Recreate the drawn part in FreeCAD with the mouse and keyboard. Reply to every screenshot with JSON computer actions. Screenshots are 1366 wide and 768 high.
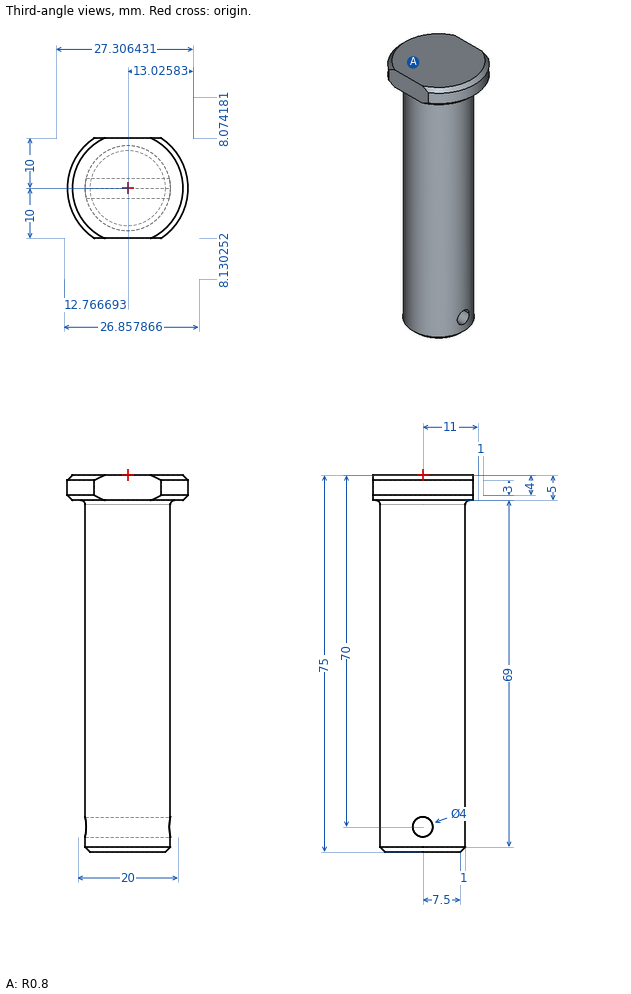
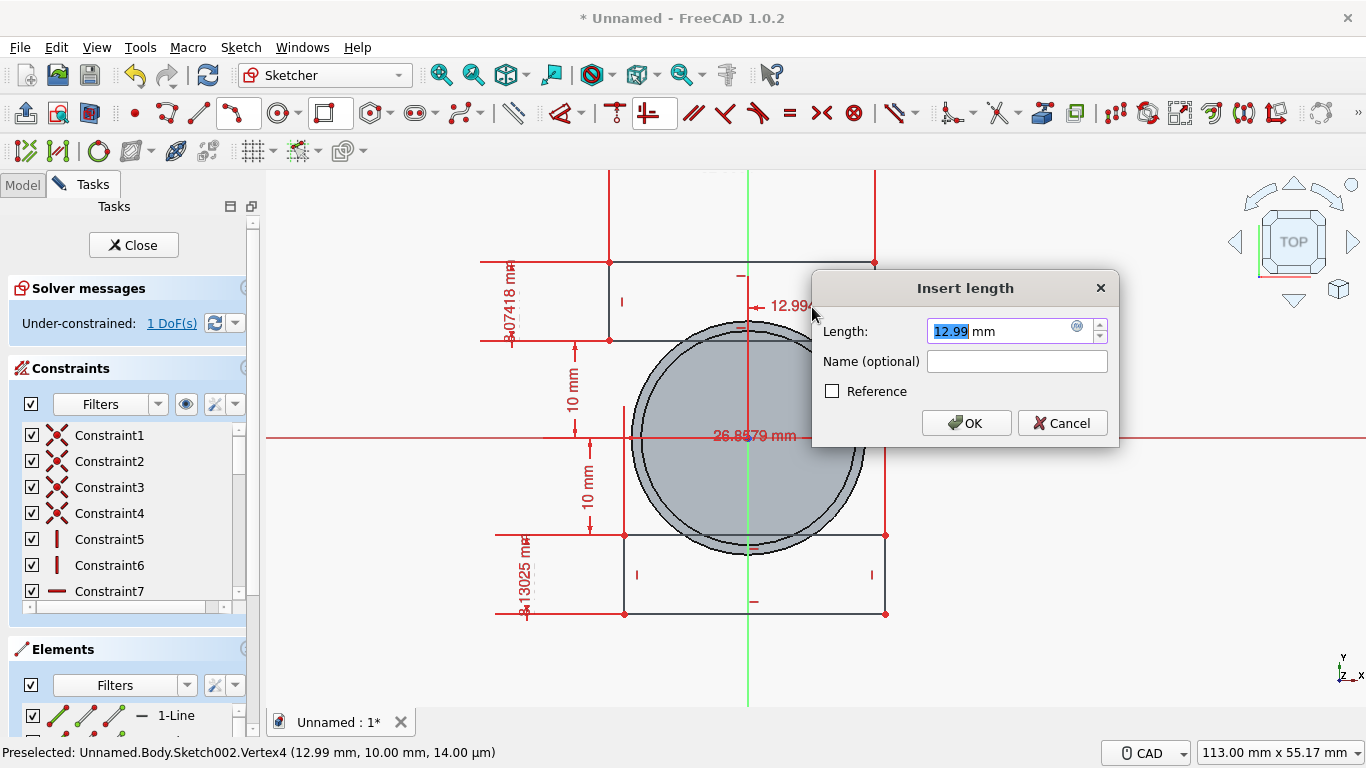
{"action": "type", "text": "13.02583"}
{"action": "key", "text": "Return"}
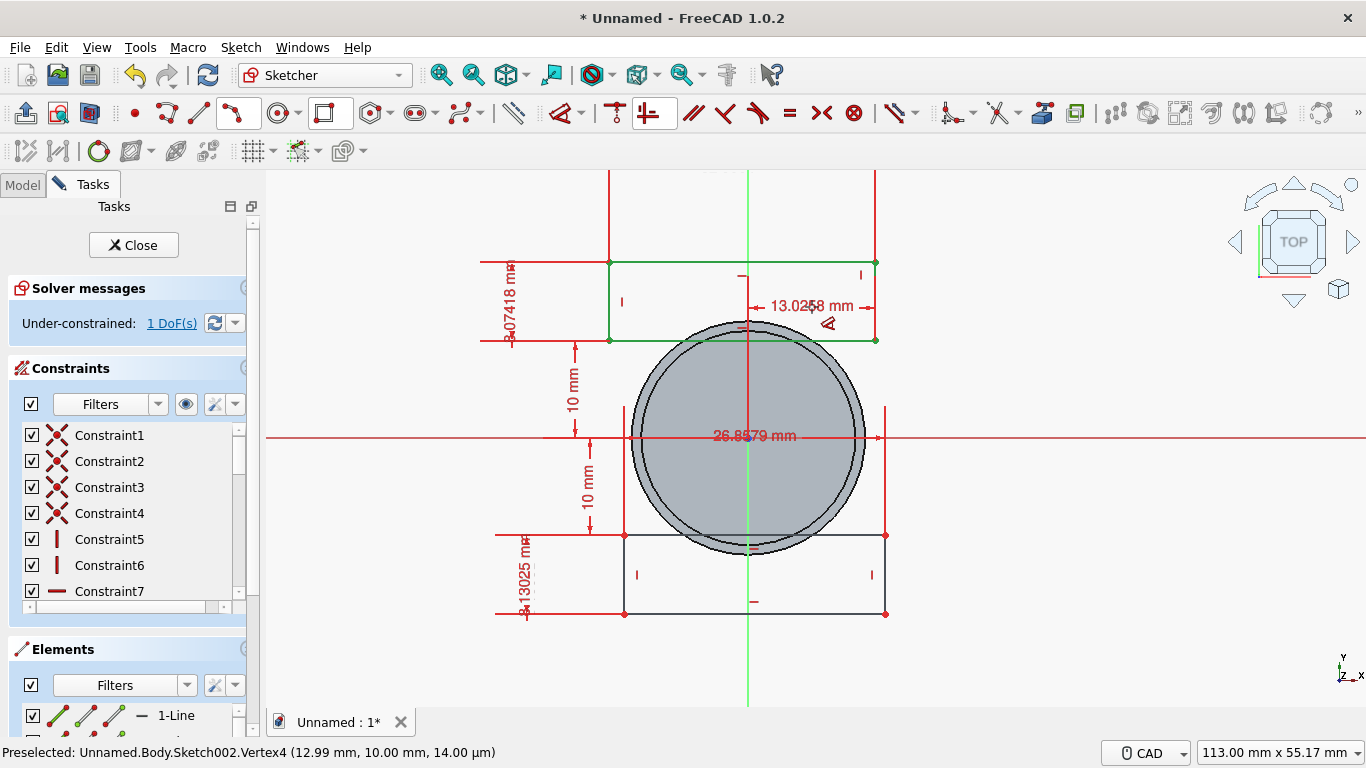
{"action": "left_click", "coordinate": [624, 535]}
{"action": "left_click", "coordinate": [686, 569]}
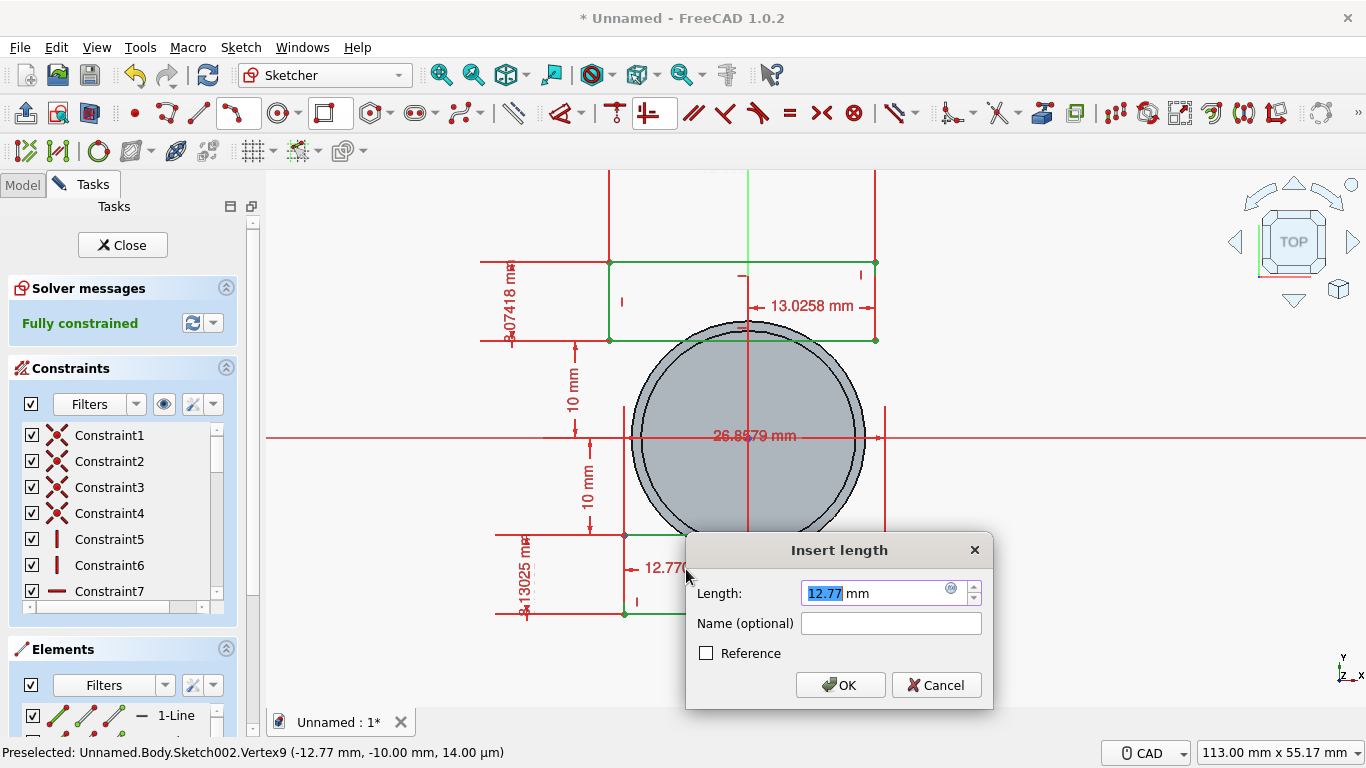
{"action": "type", "text": "12.766693"}
{"action": "key", "text": "Return"}
{"action": "key", "text": "Escape"}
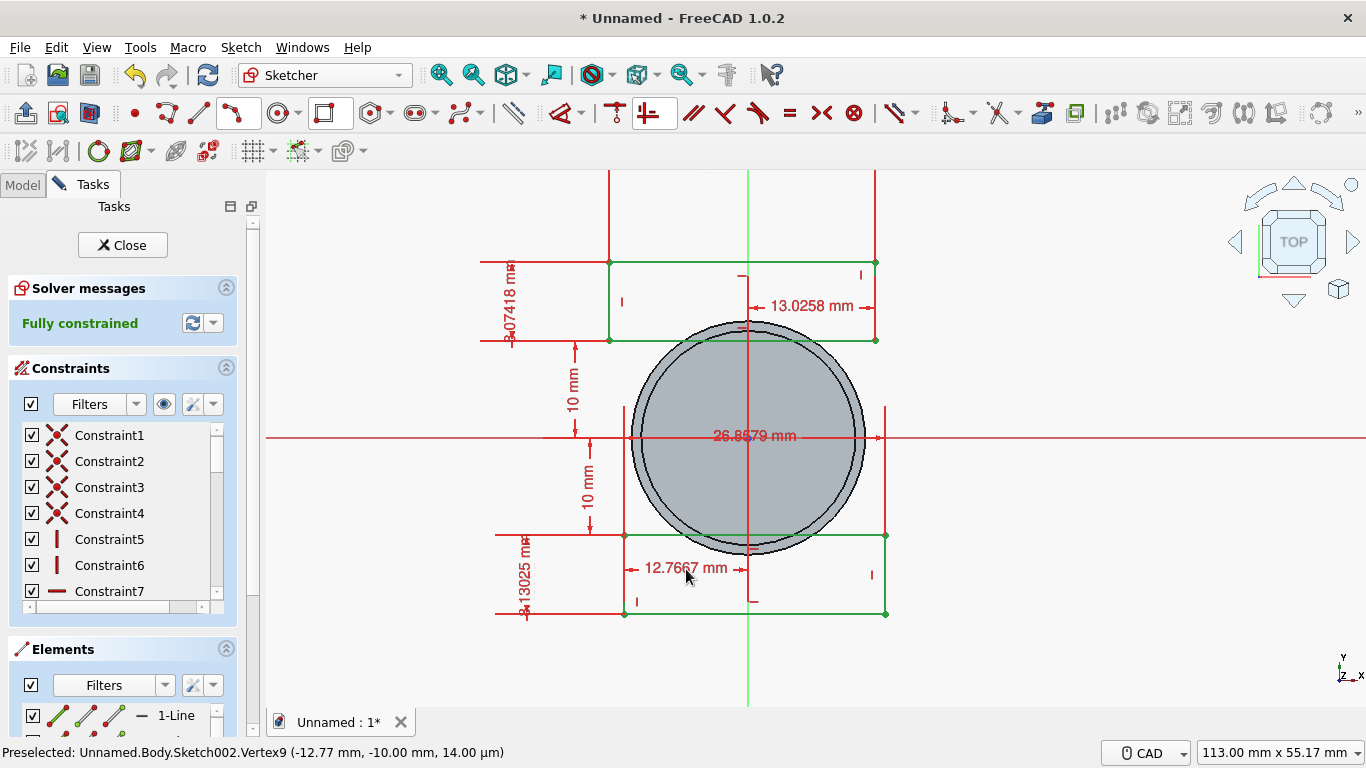
{"action": "left_click", "coordinate": [123, 245]}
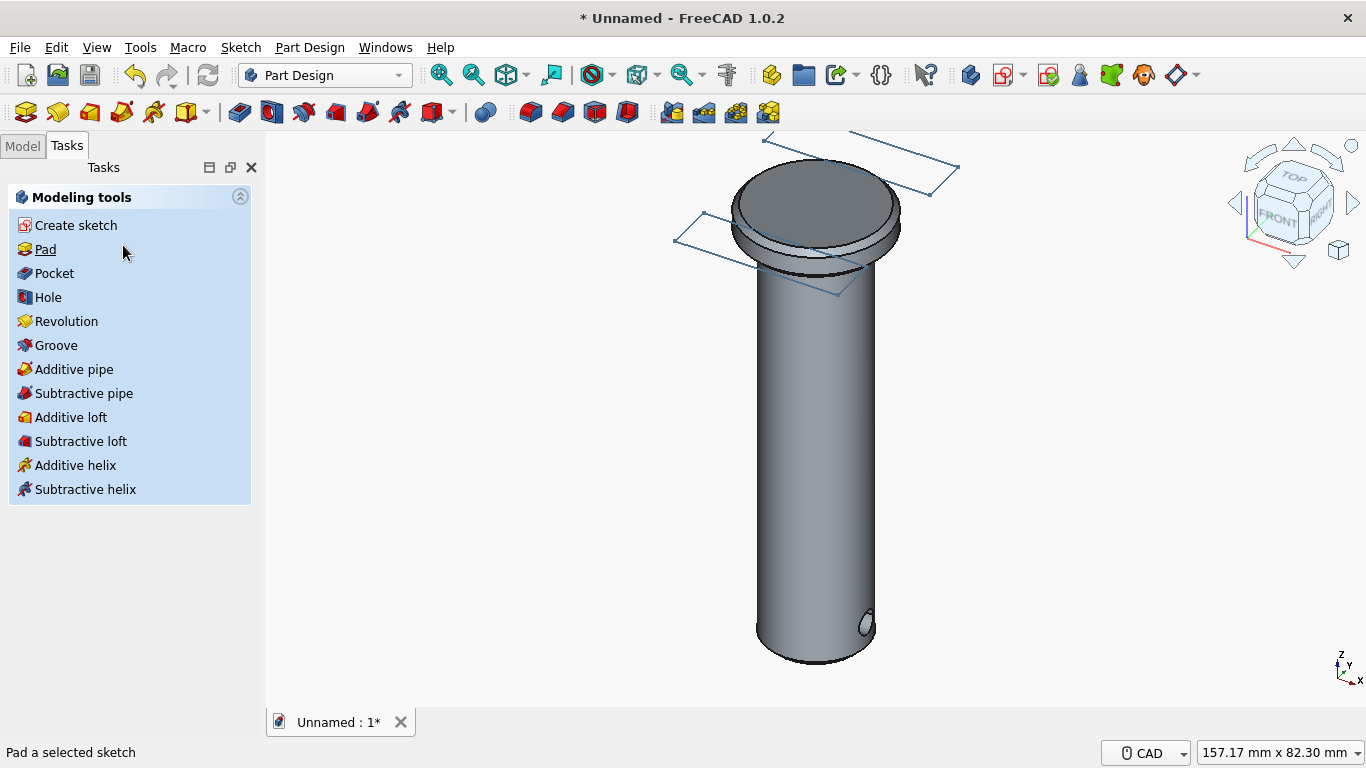
{"action": "left_click", "coordinate": [240, 112]}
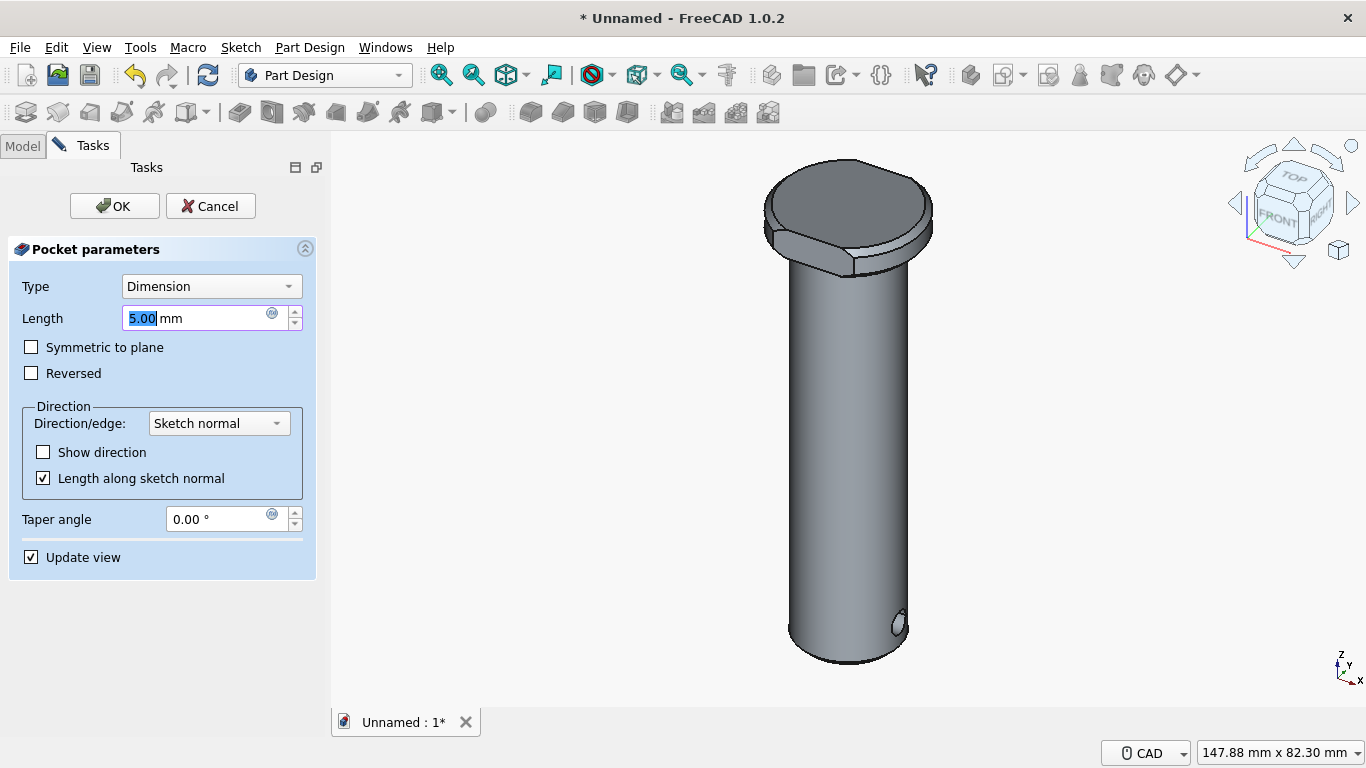
{"action": "type", "text": "10"}
{"action": "key", "text": "Tab"}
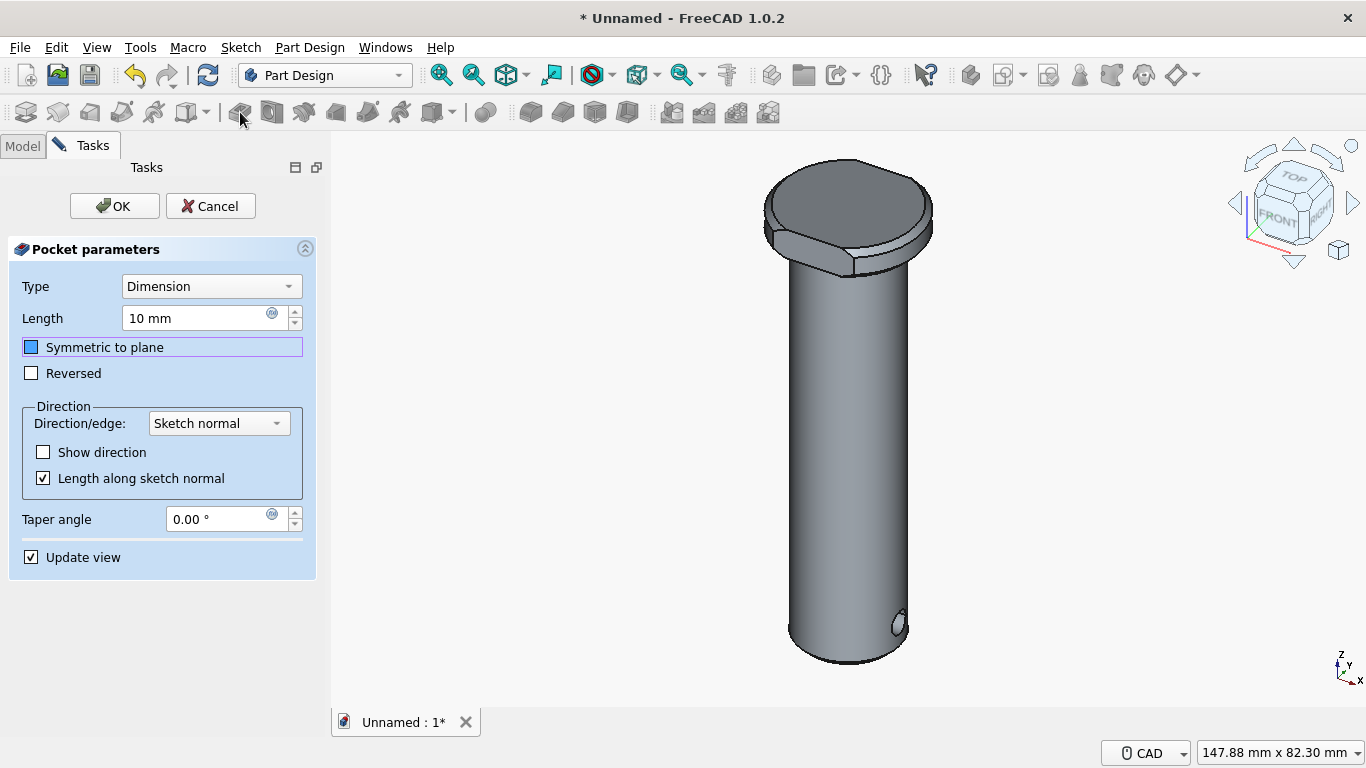
{"action": "left_click", "coordinate": [30, 347]}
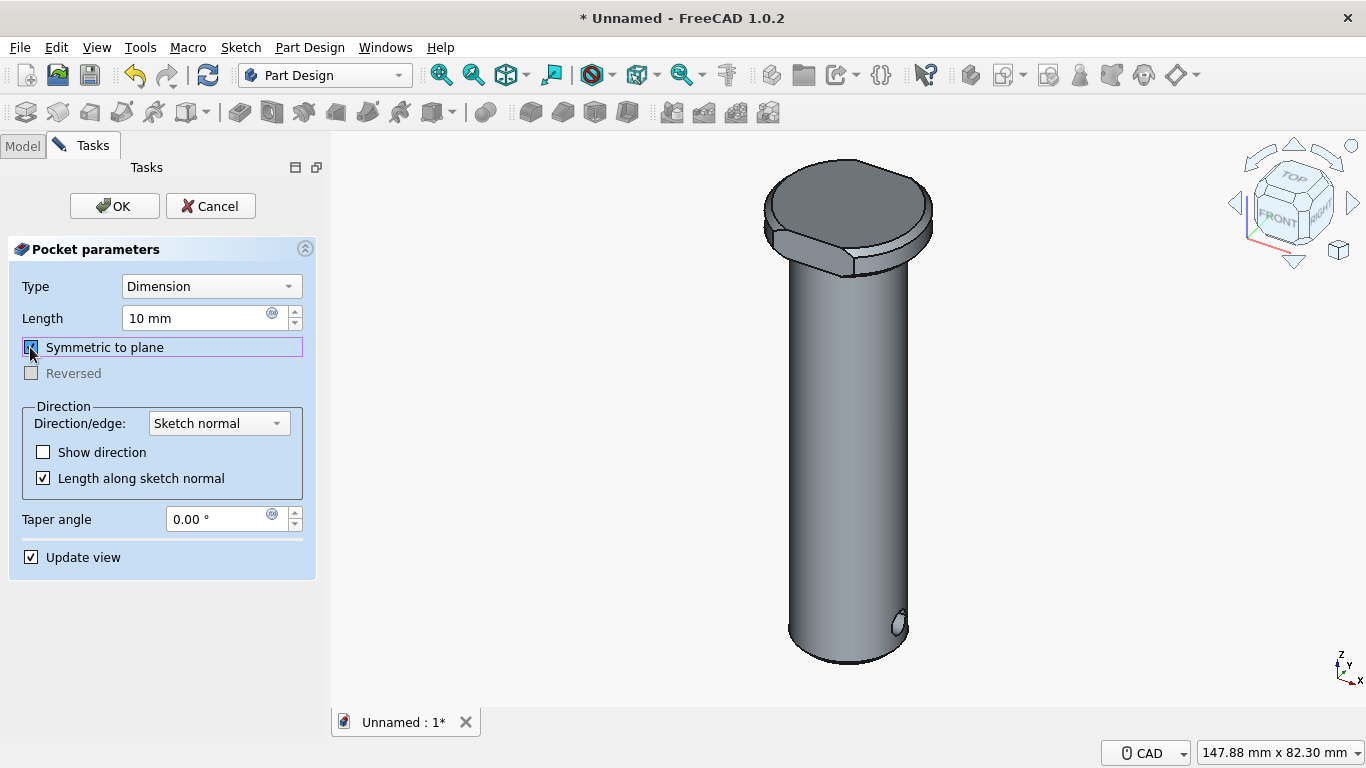
{"action": "left_click", "coordinate": [115, 206]}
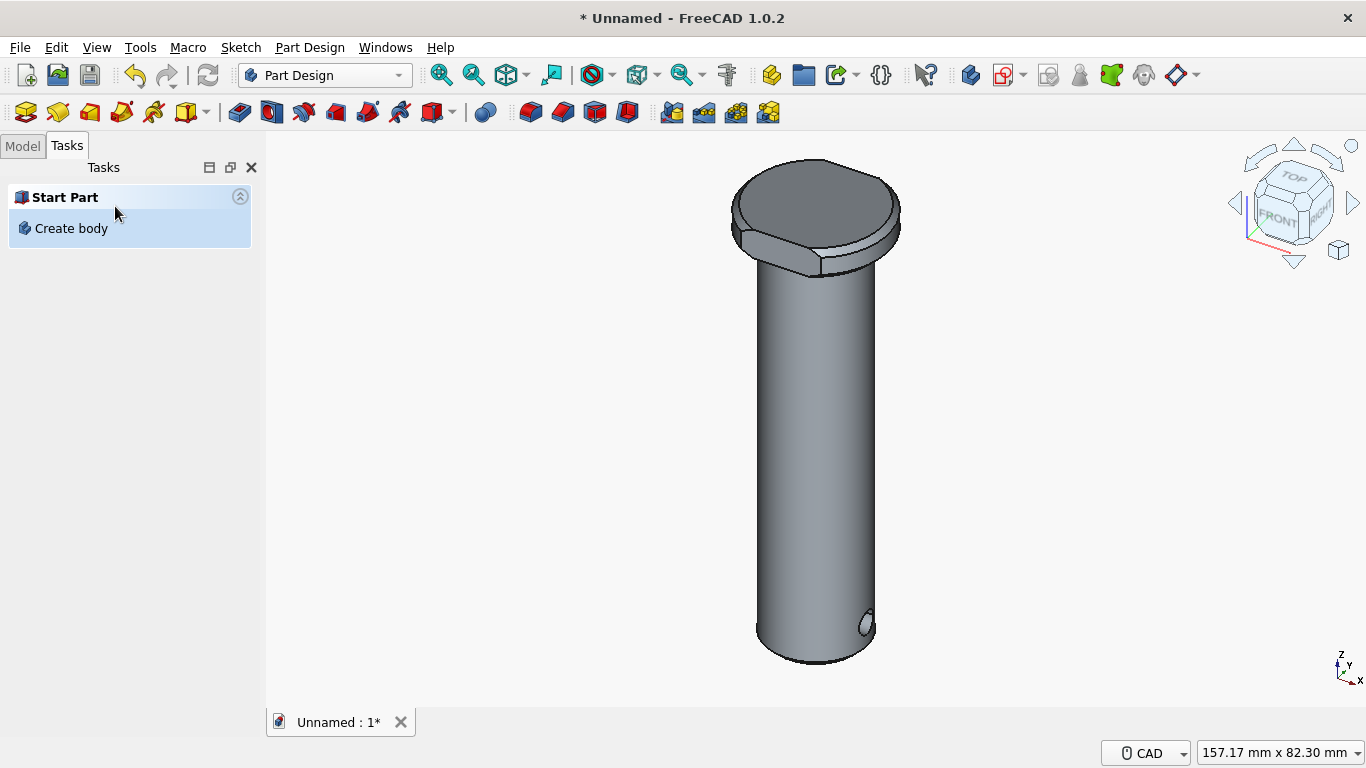
{"action": "key", "text": "0"}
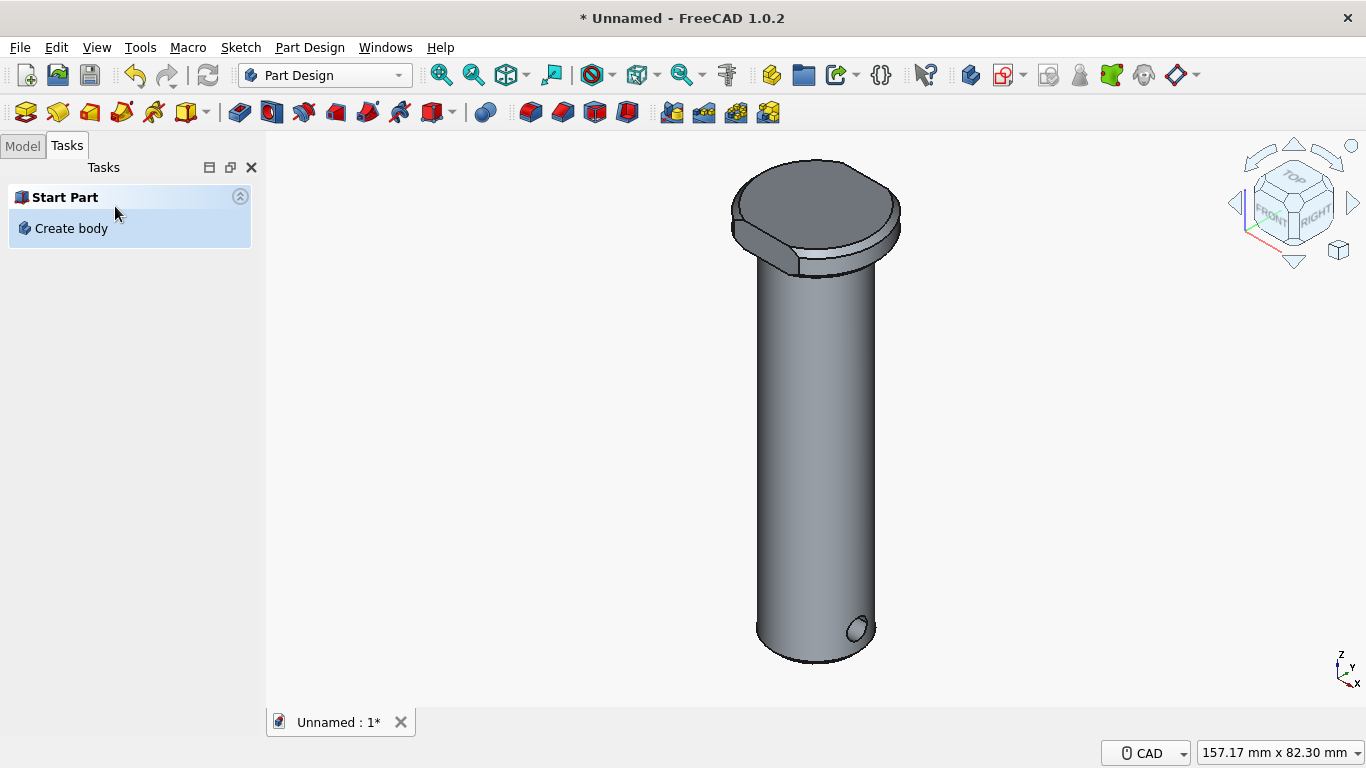
{"action": "key", "text": "2"}